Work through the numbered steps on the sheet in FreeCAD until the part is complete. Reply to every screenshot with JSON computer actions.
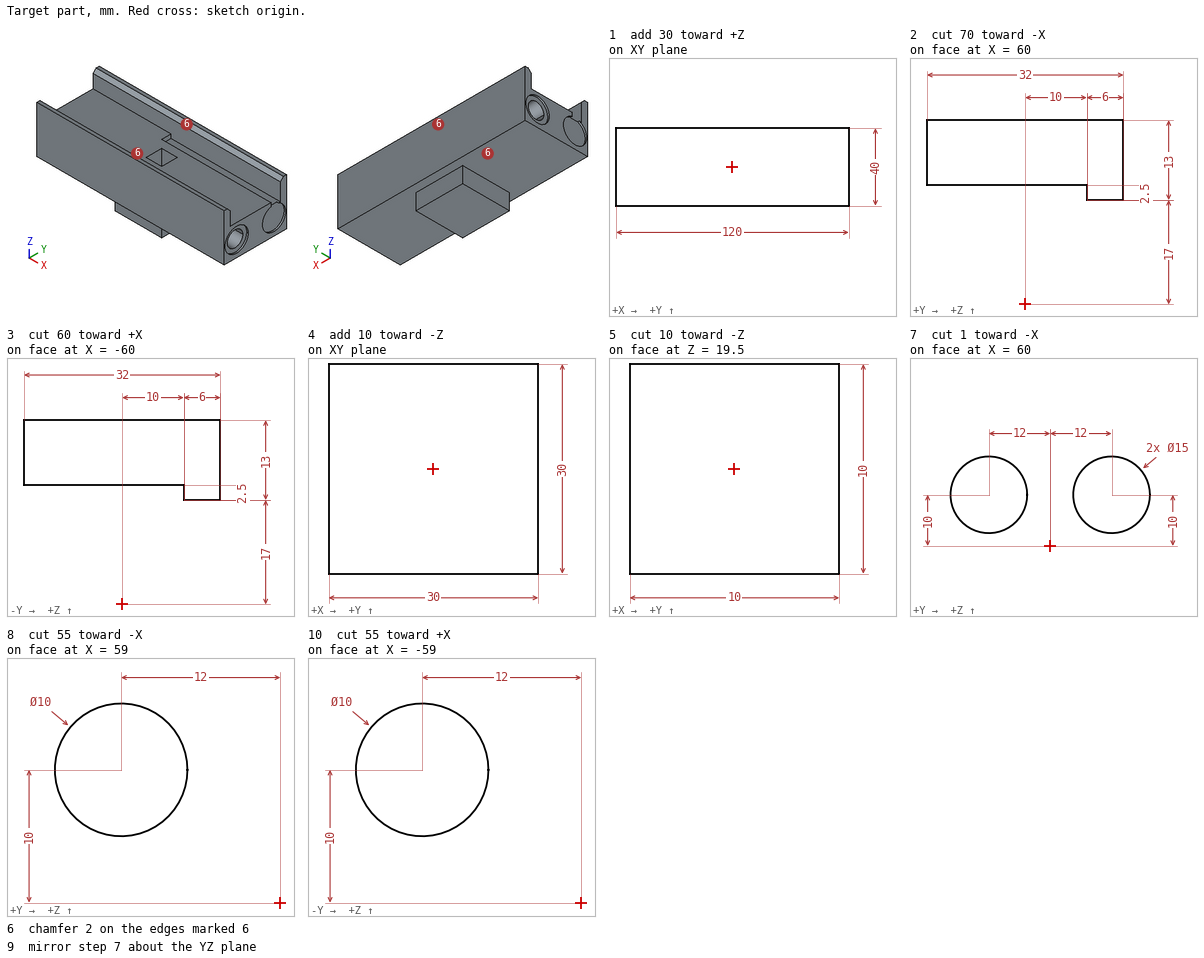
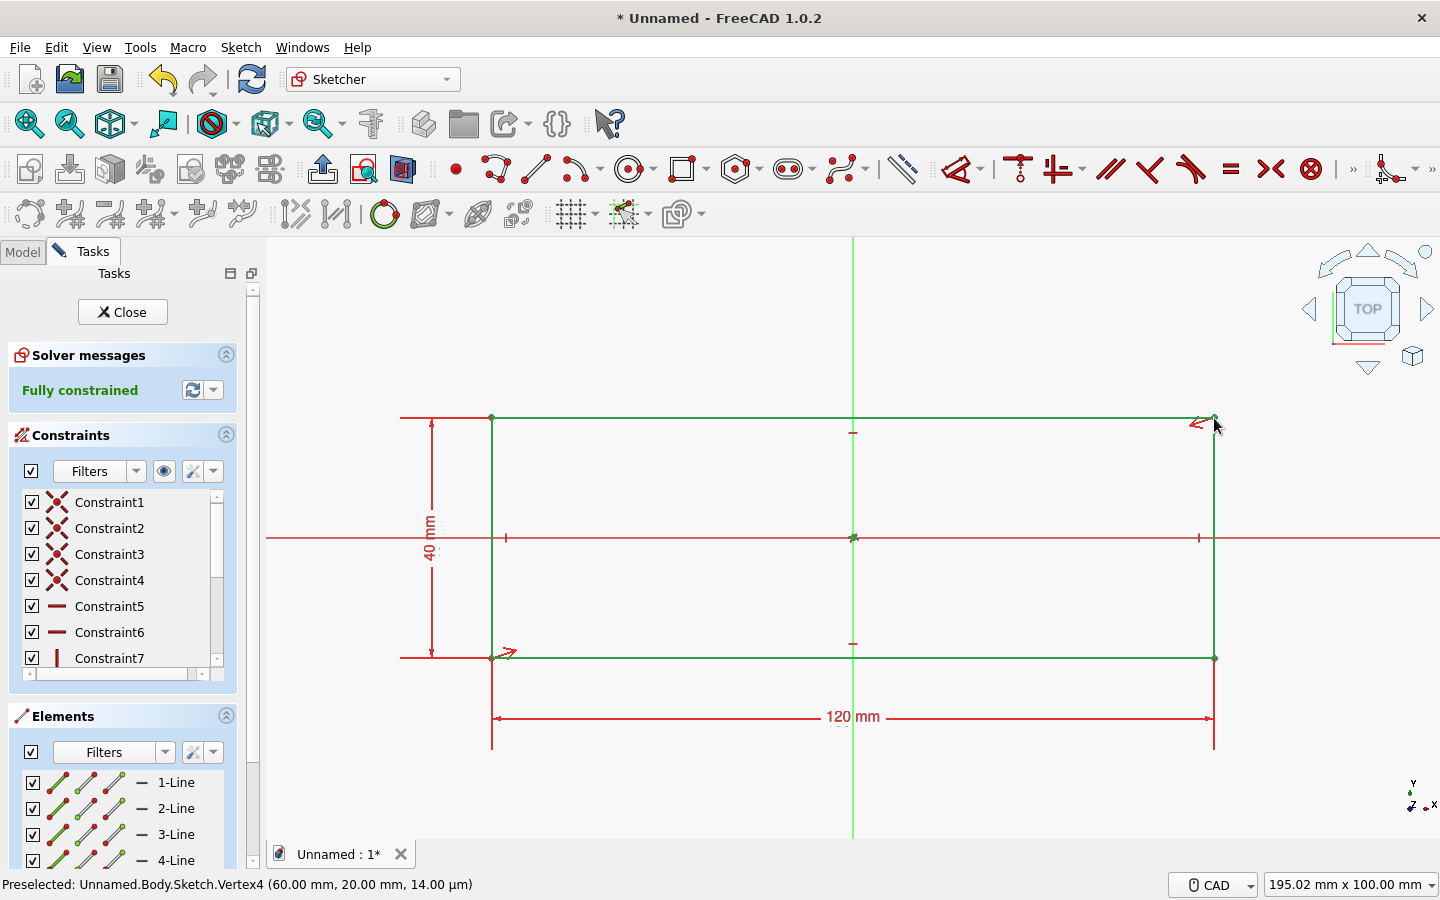
{"action": "left_click", "coordinate": [123, 312]}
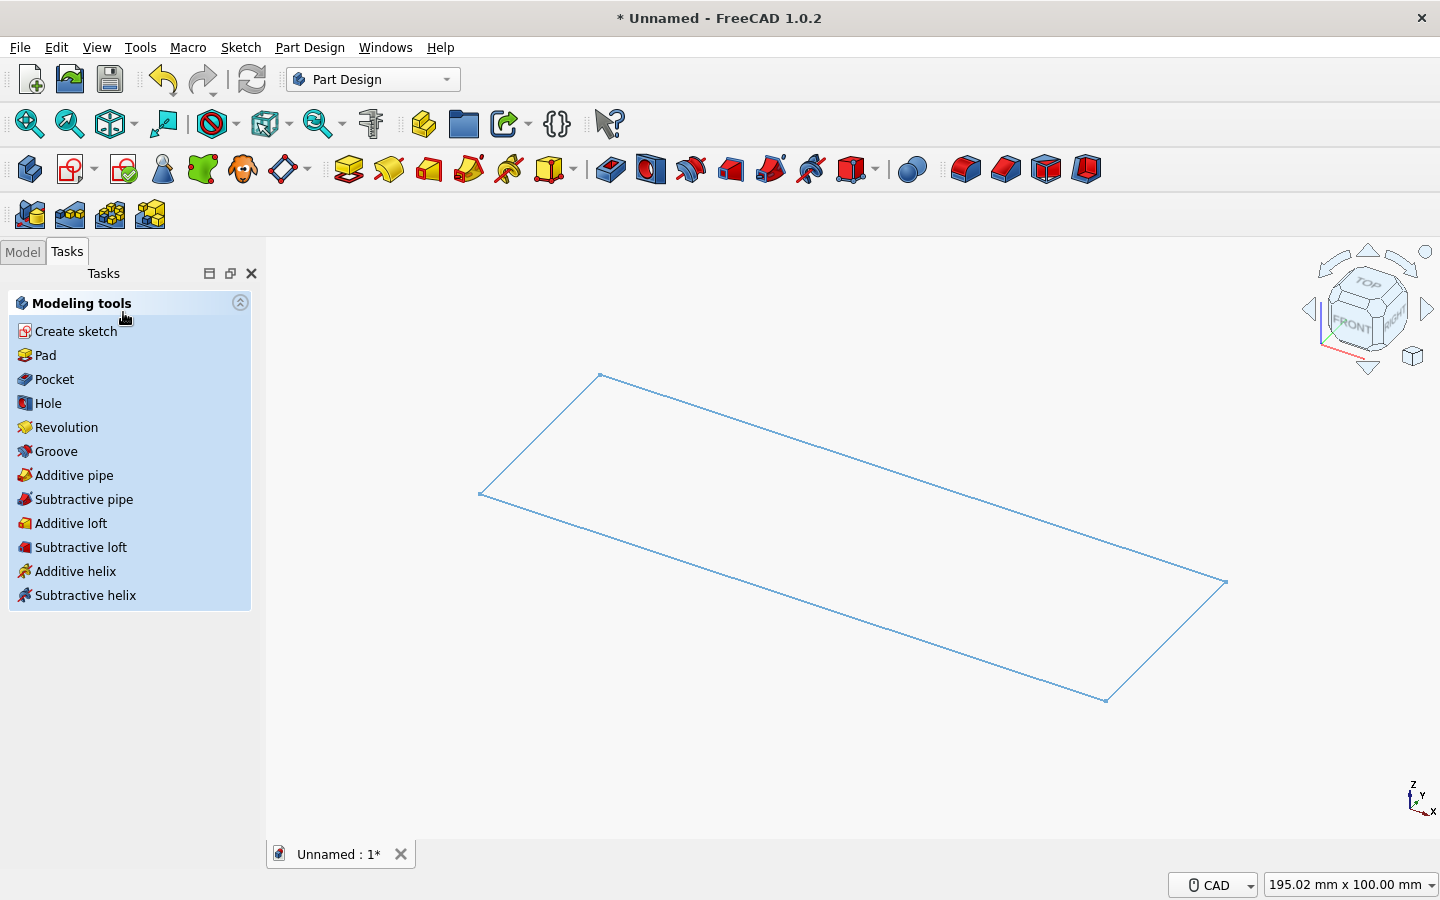
{"action": "left_click", "coordinate": [350, 170]}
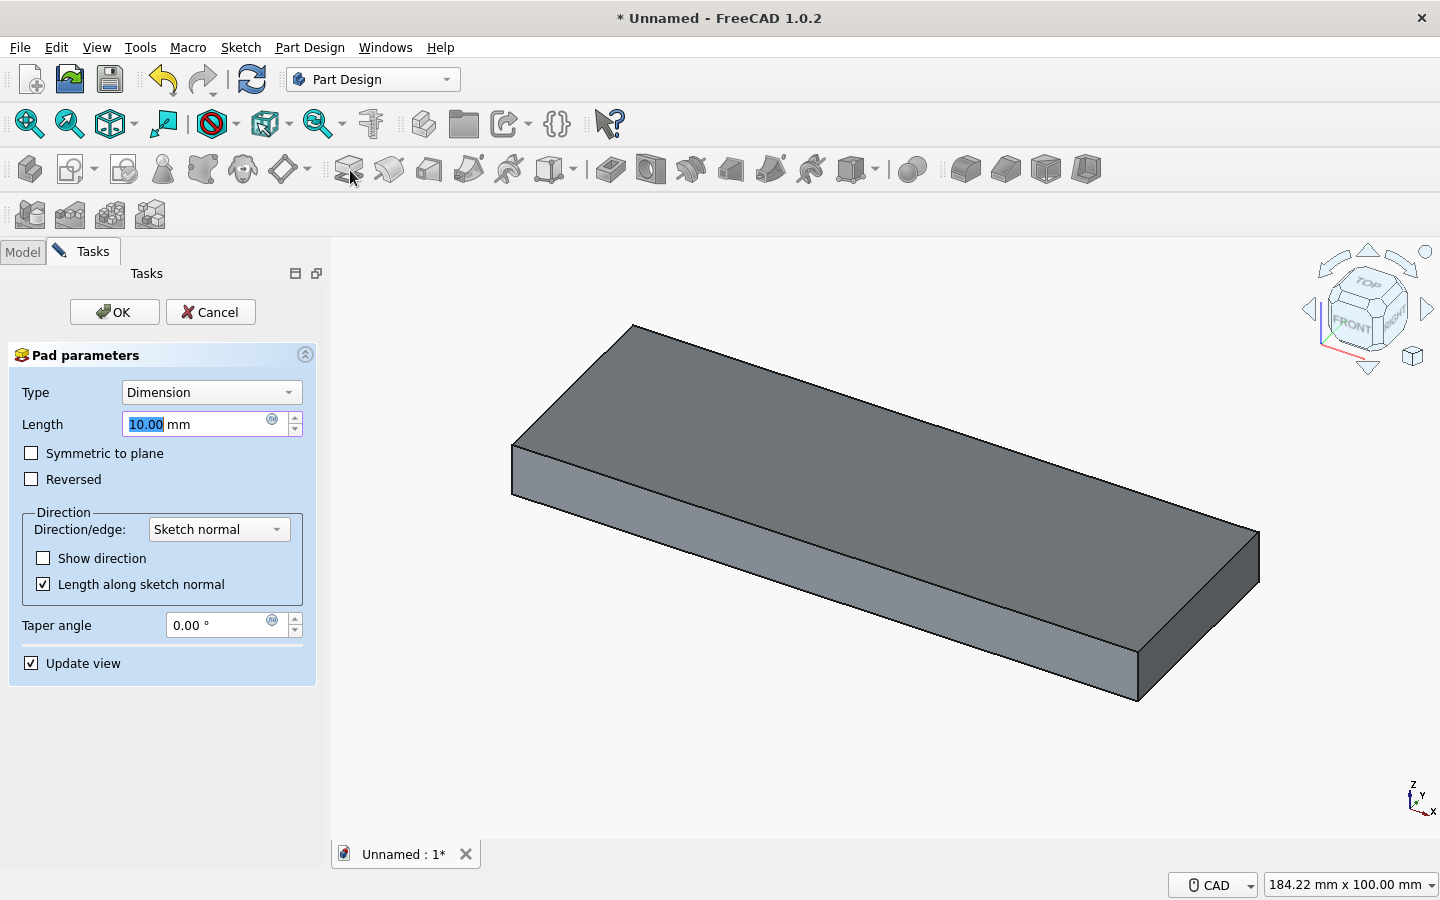
{"action": "type", "text": "30"}
{"action": "key", "text": "Tab"}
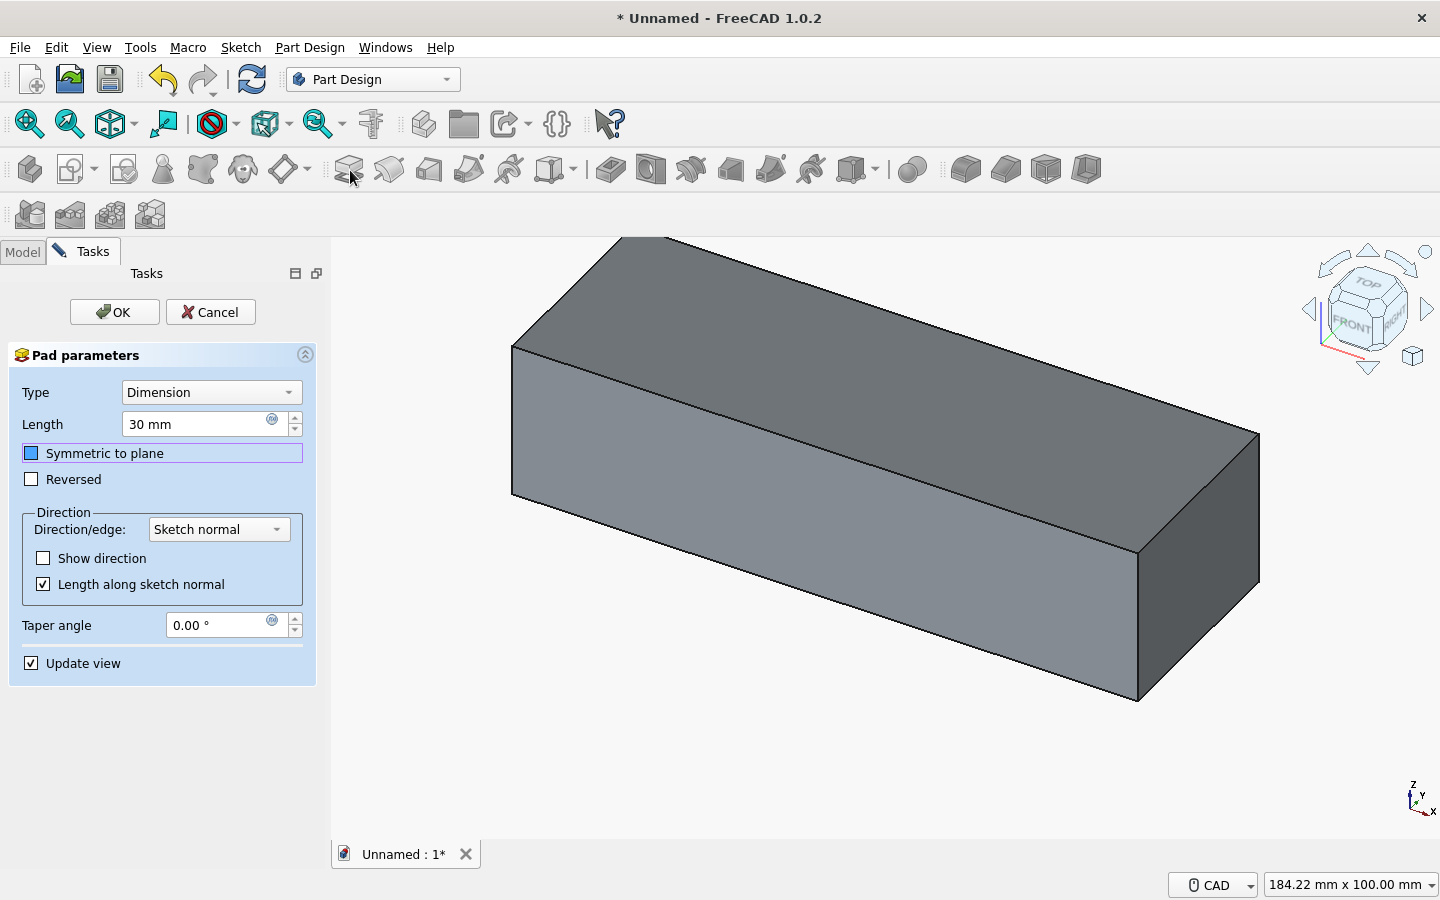
{"action": "left_click", "coordinate": [115, 312]}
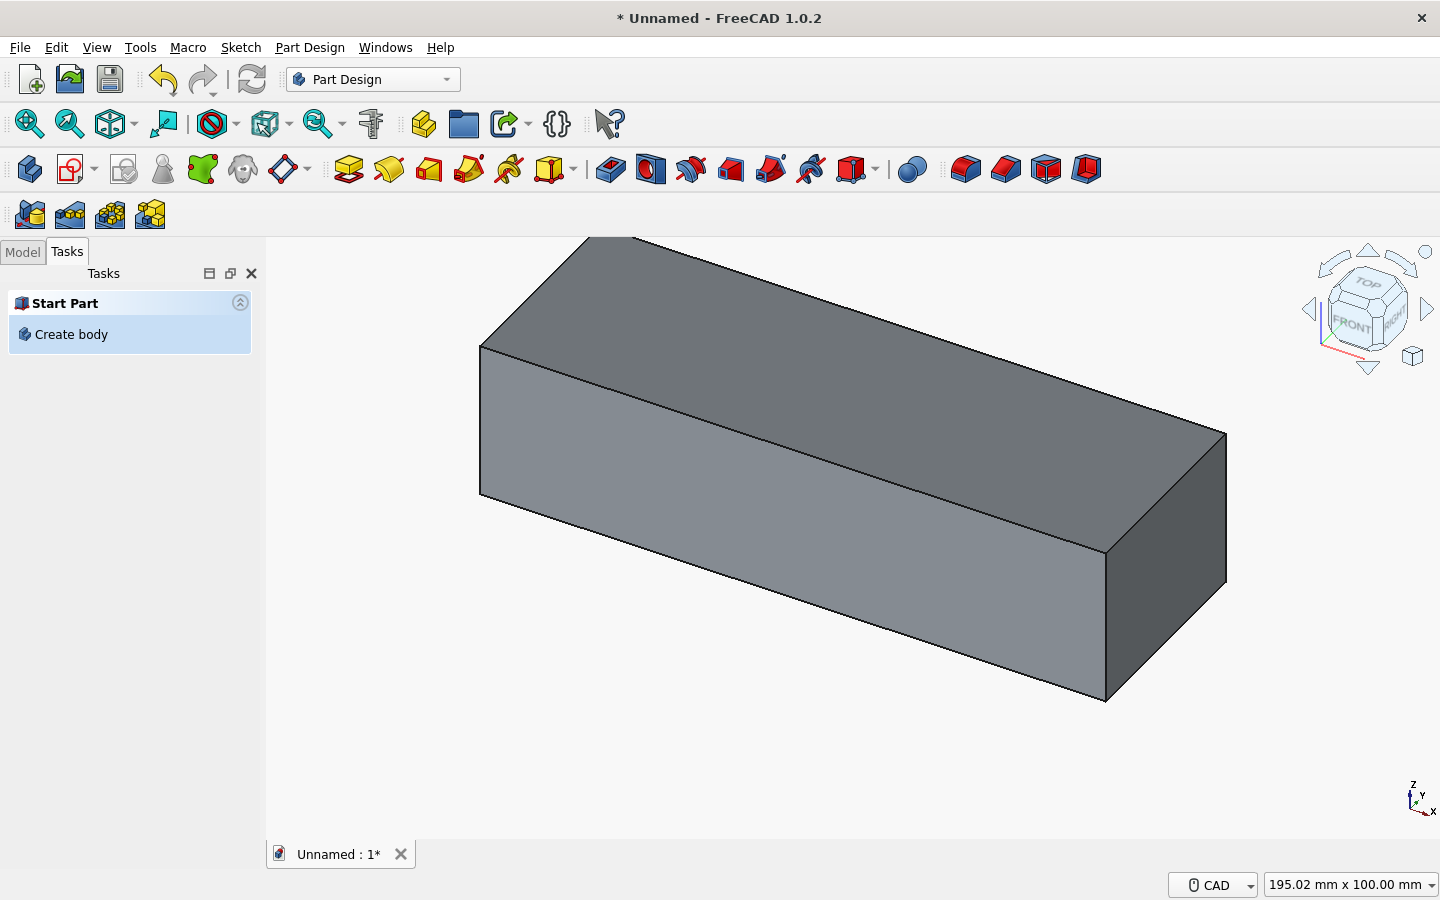
{"action": "key", "text": "v f"}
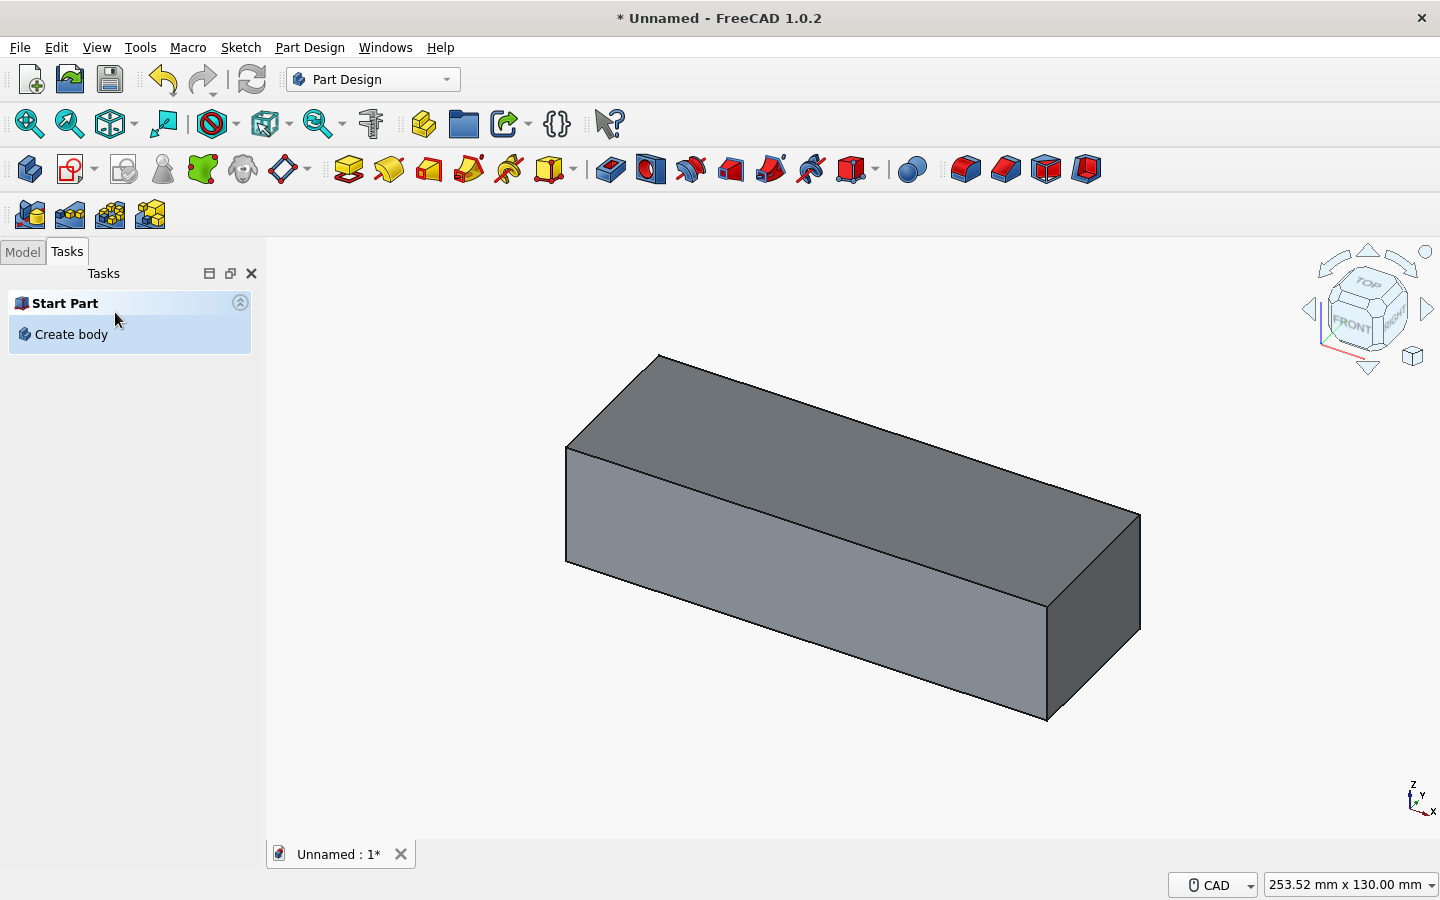
{"action": "left_click", "coordinate": [1094, 617]}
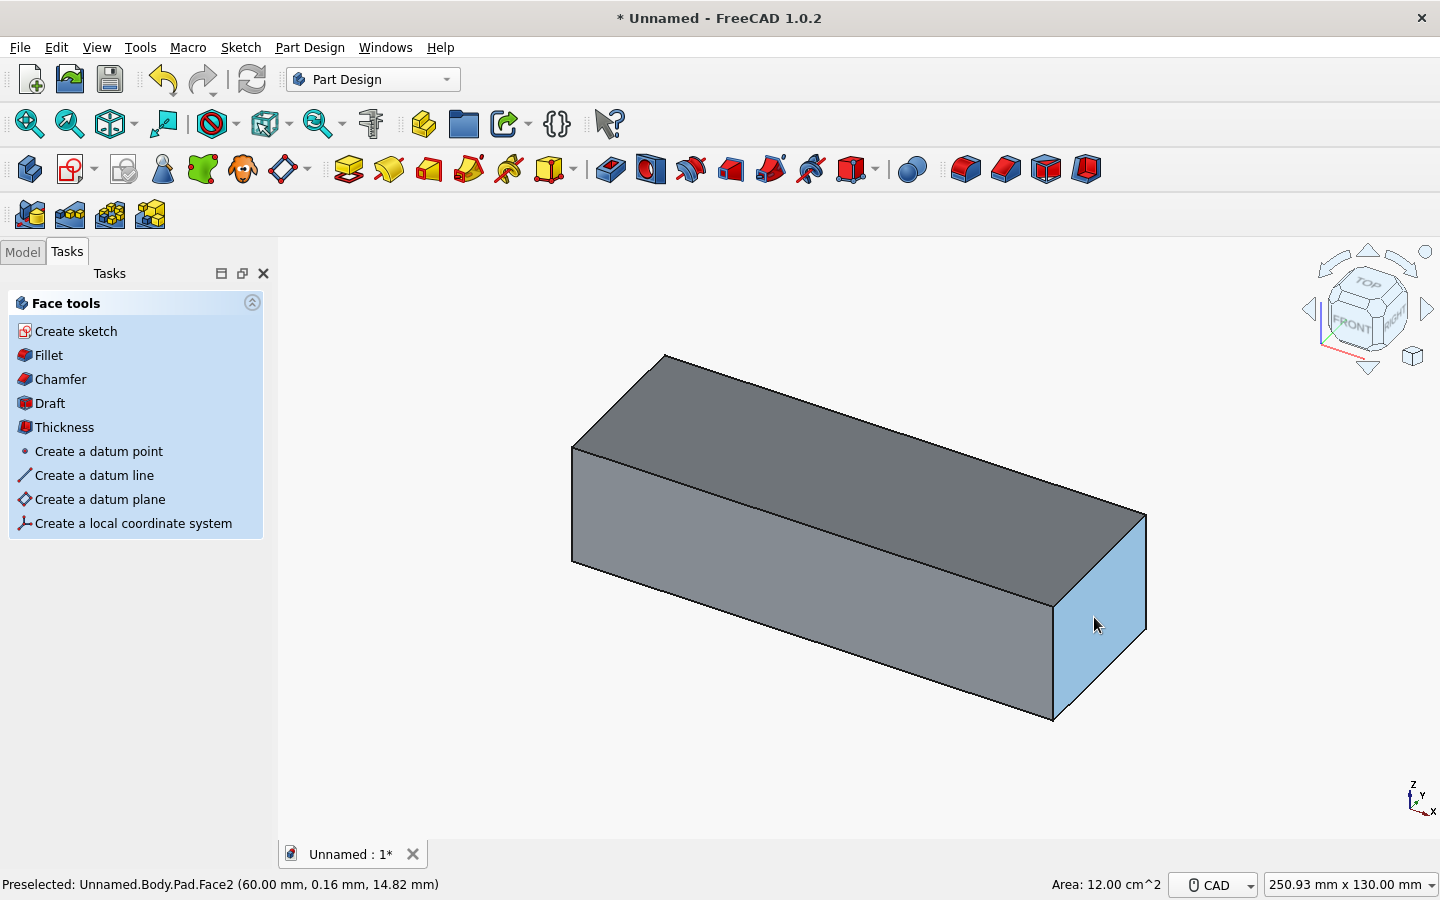
{"action": "left_click", "coordinate": [70, 170]}